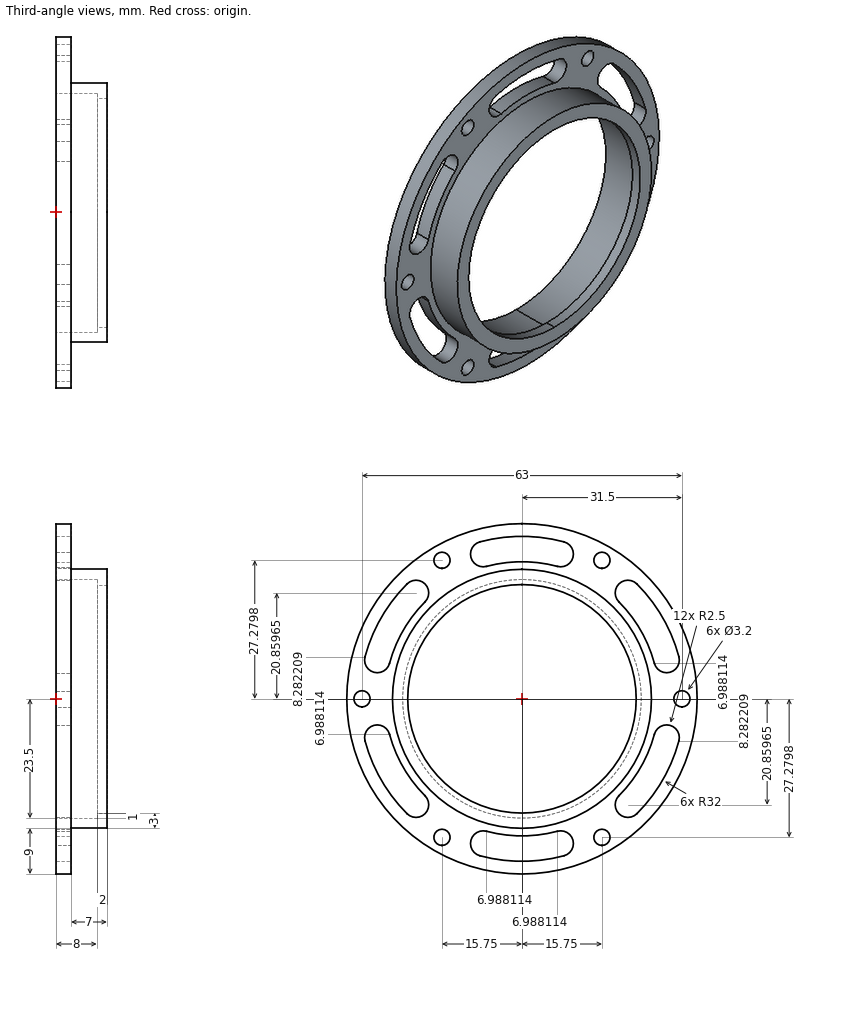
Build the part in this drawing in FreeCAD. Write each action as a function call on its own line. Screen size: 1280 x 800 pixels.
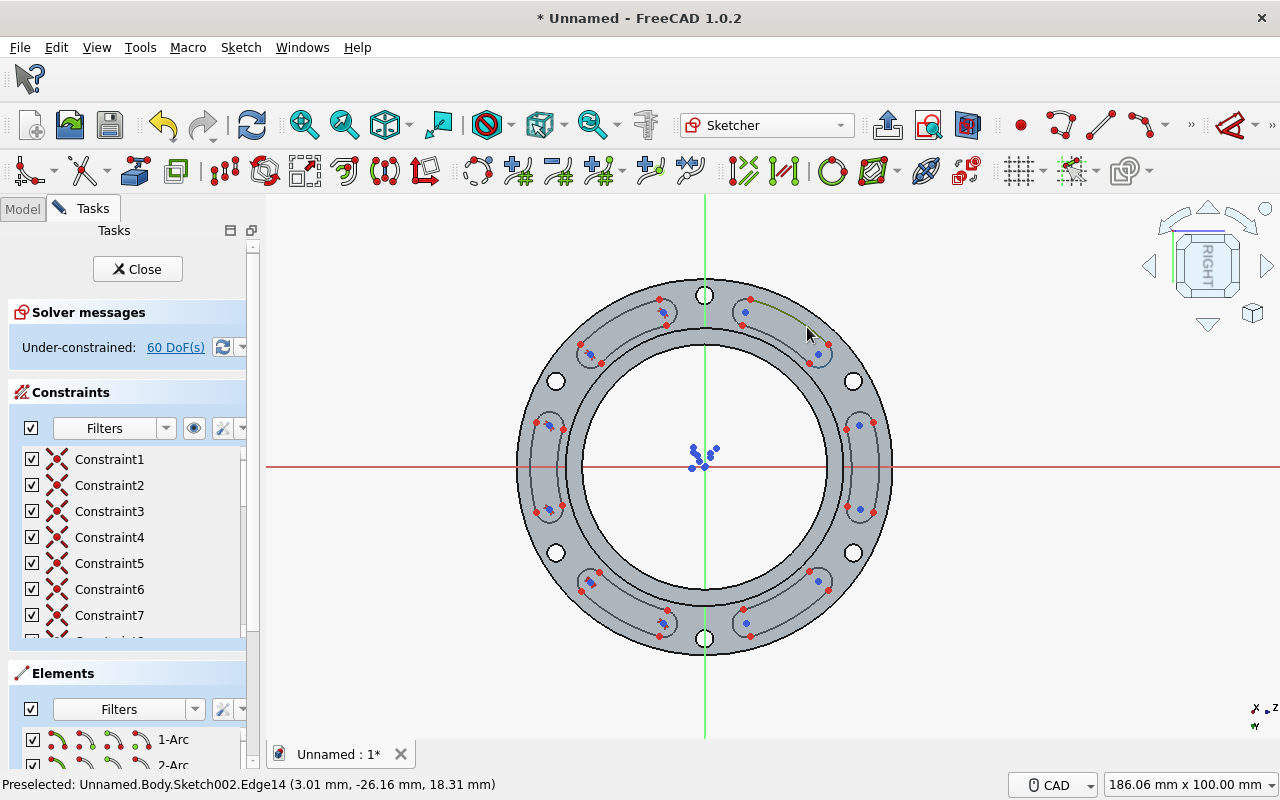
key(t)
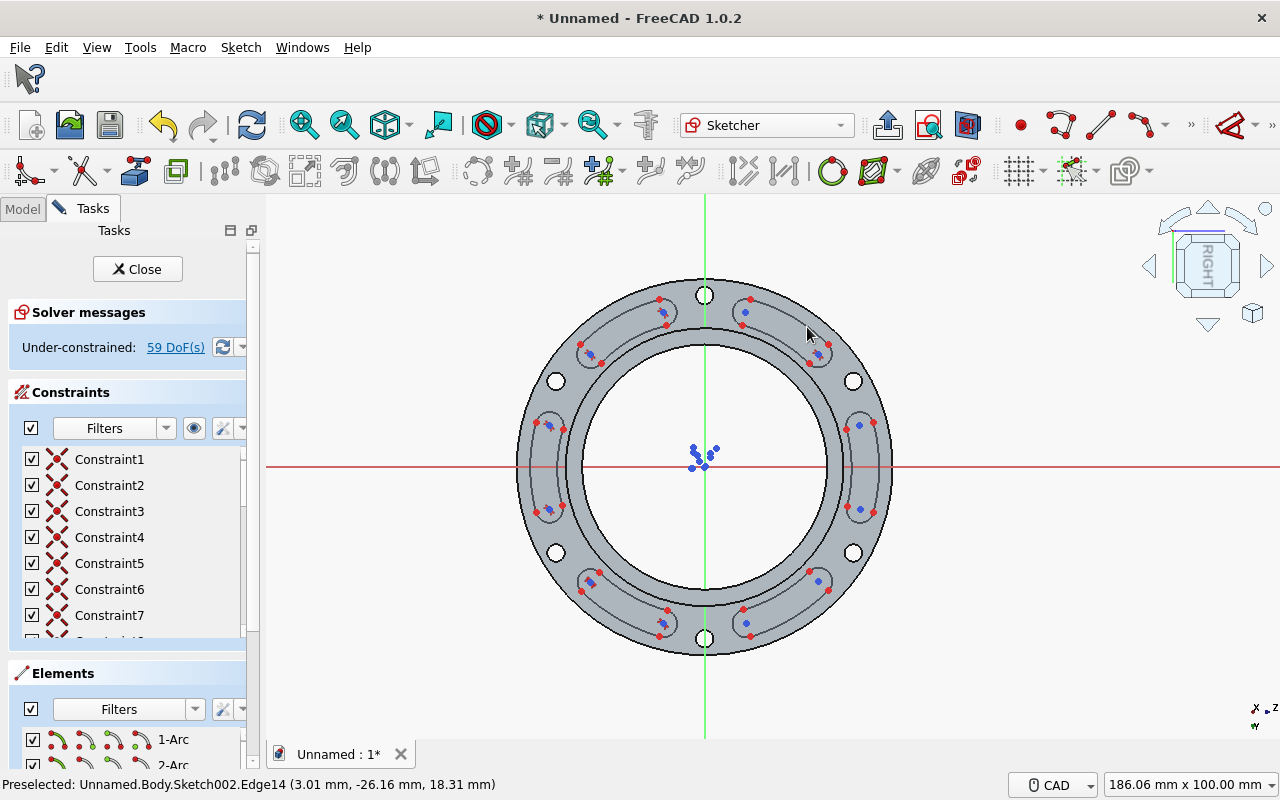
click(821, 367)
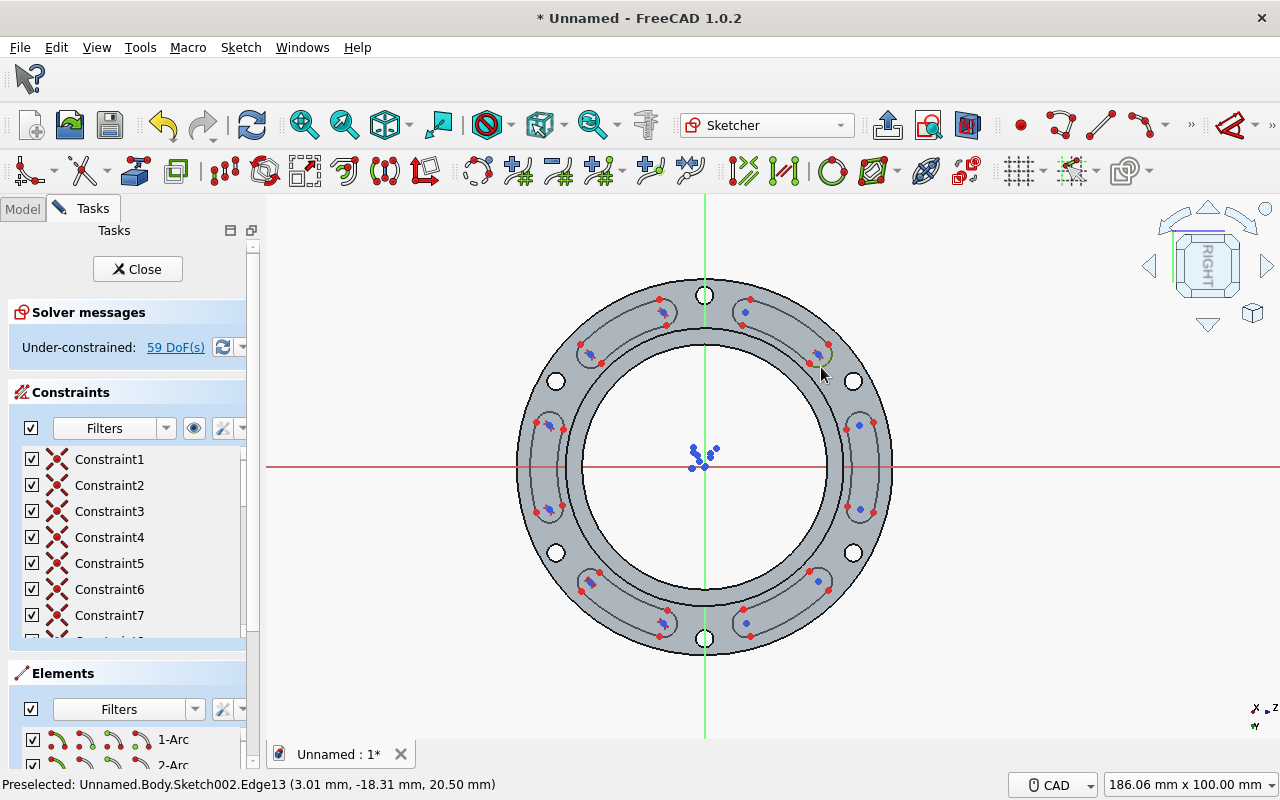
click(791, 349)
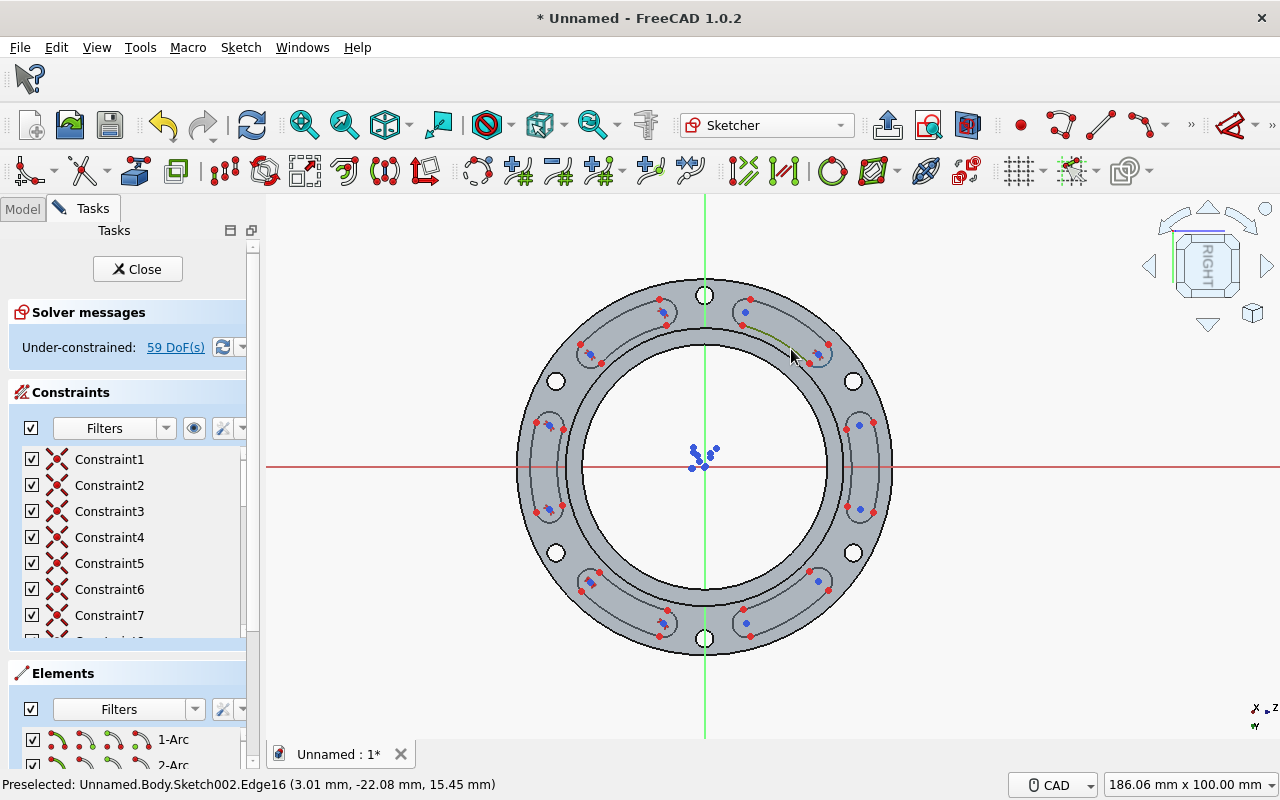
key(t)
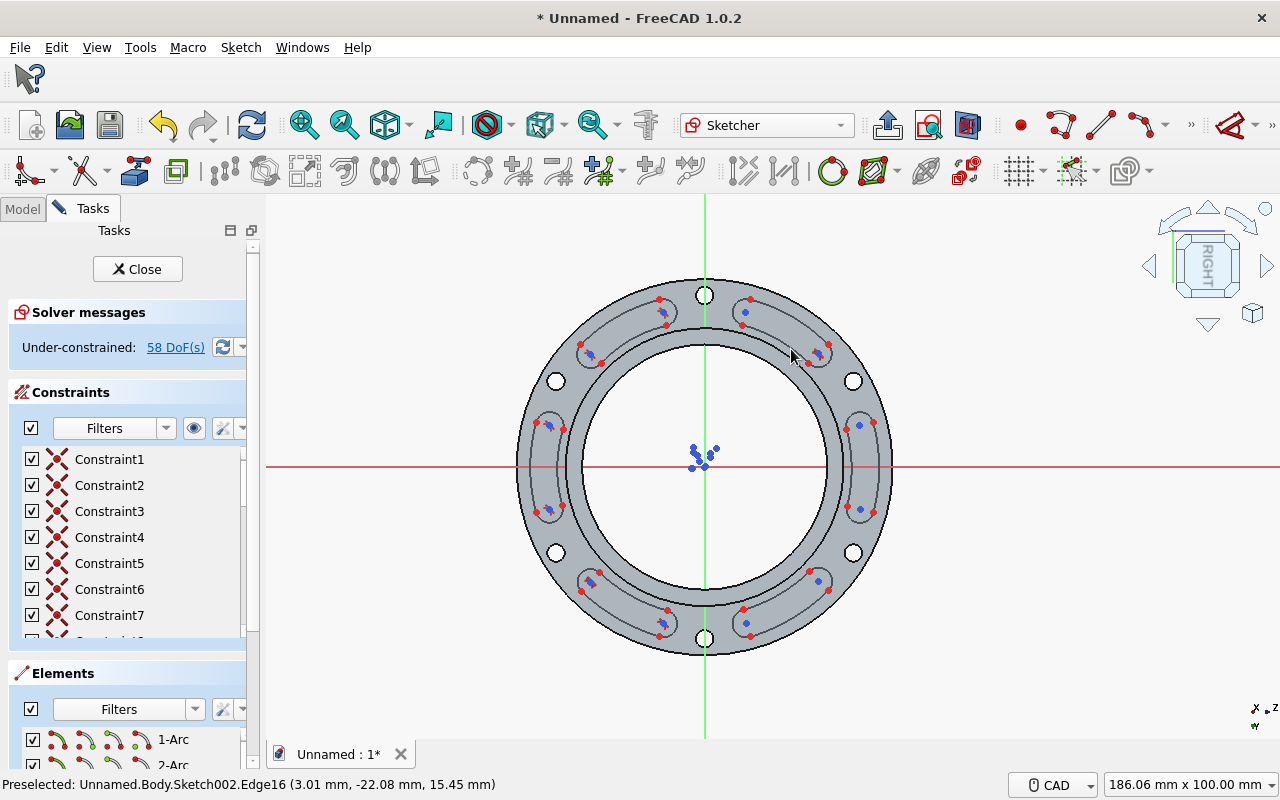
click(807, 327)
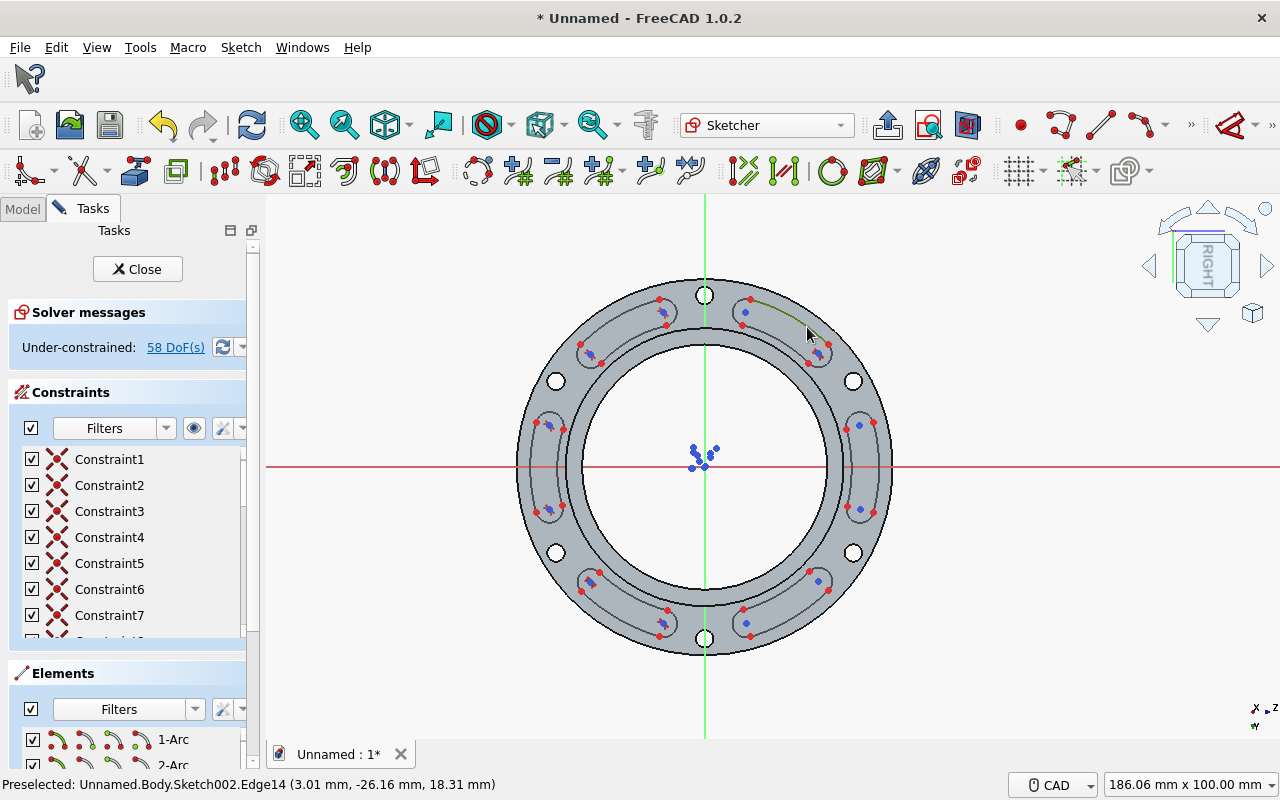
click(738, 302)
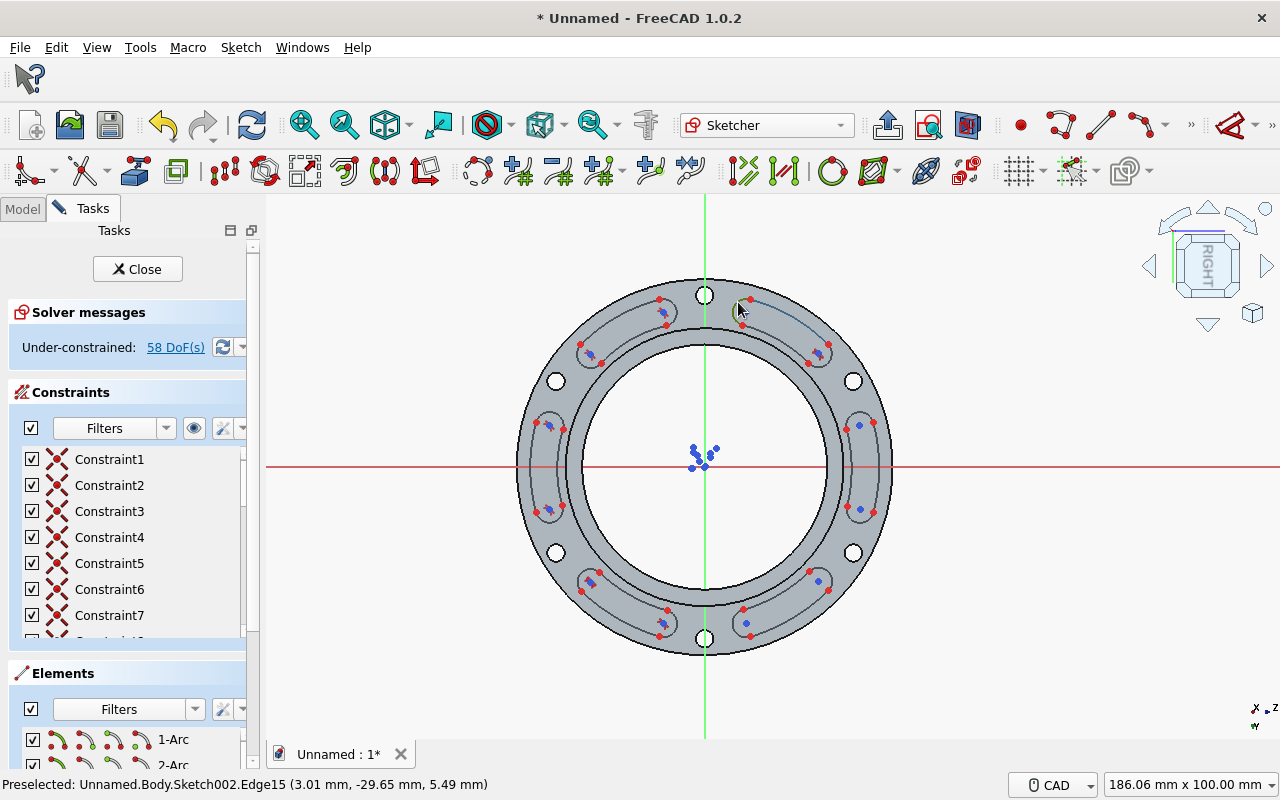
key(t)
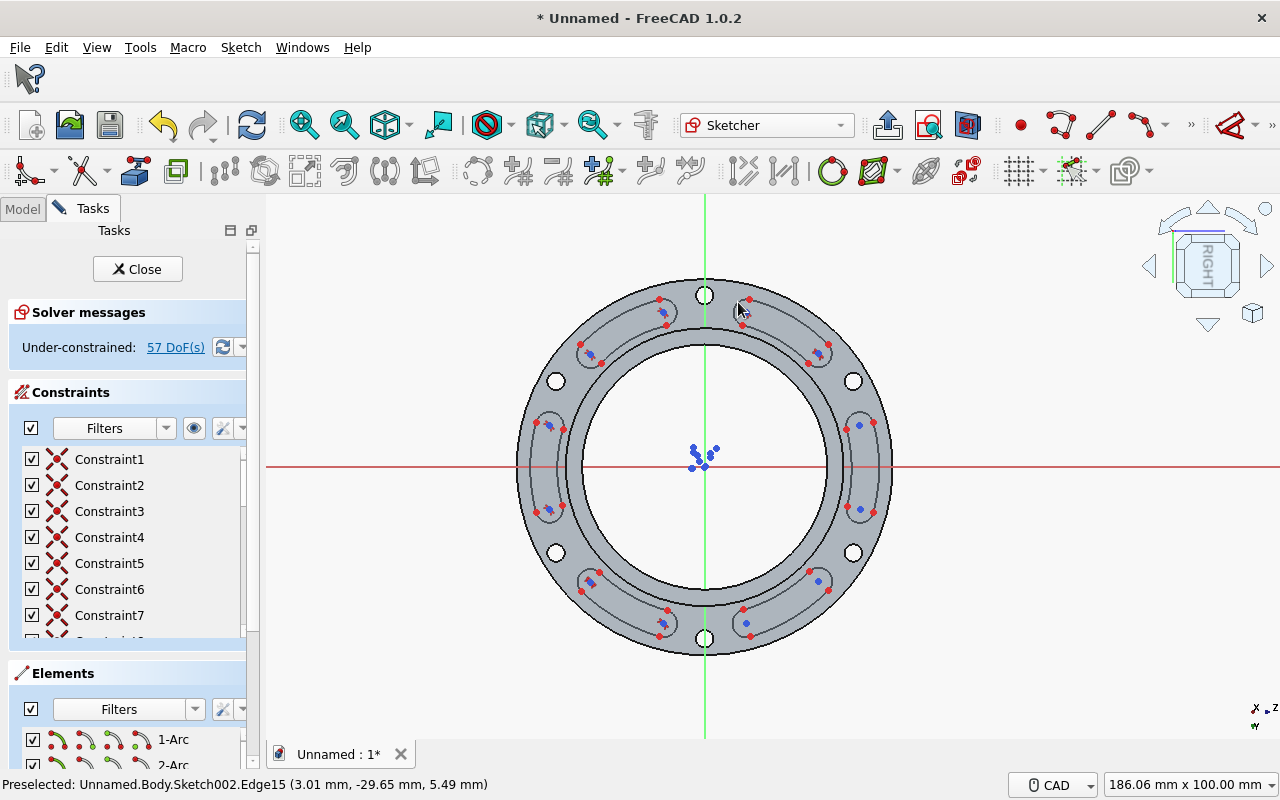
click(738, 302)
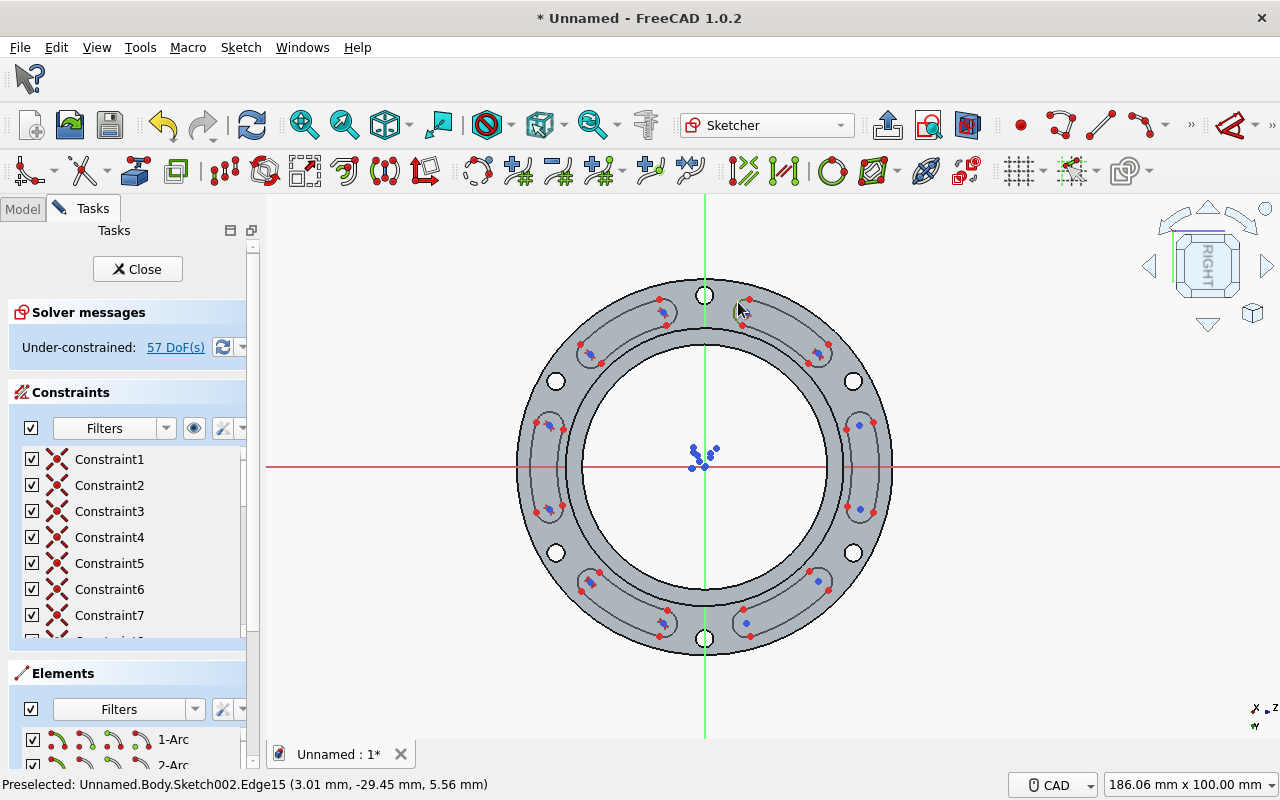
click(791, 348)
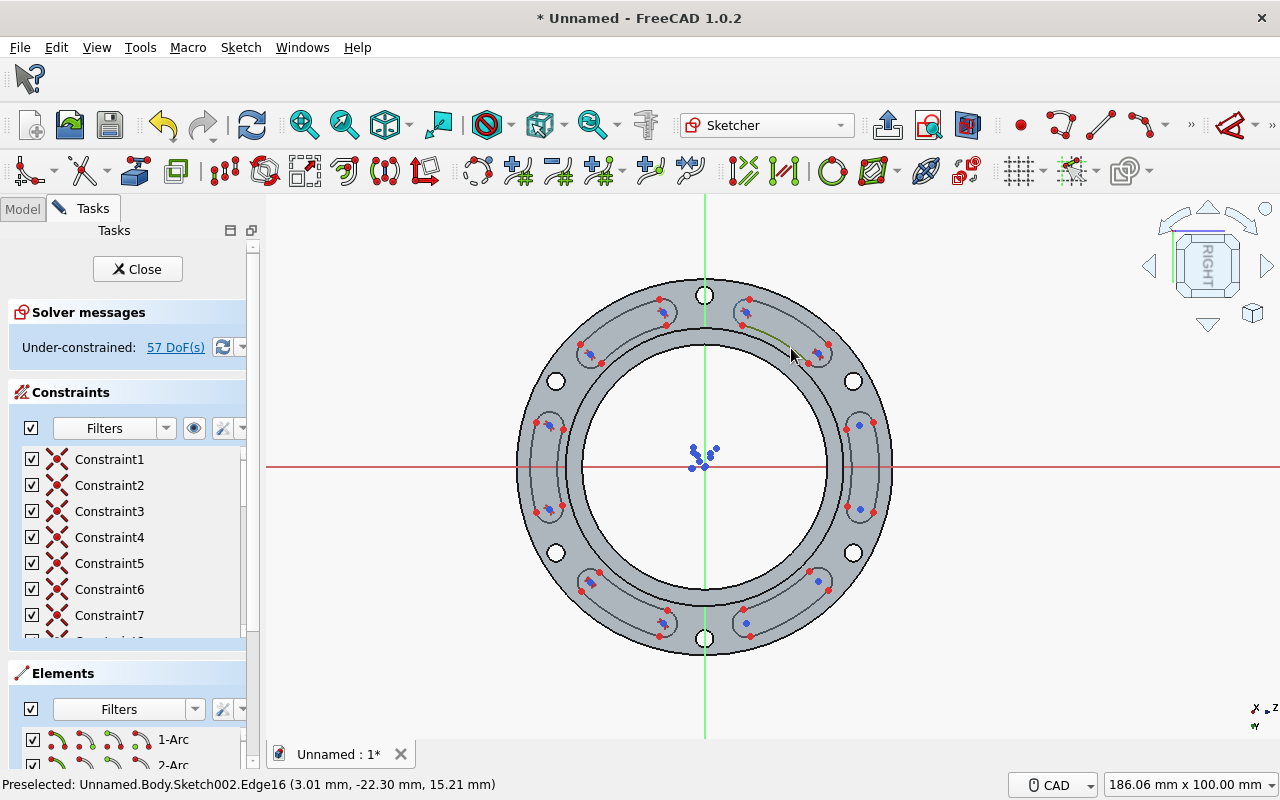
key(t)